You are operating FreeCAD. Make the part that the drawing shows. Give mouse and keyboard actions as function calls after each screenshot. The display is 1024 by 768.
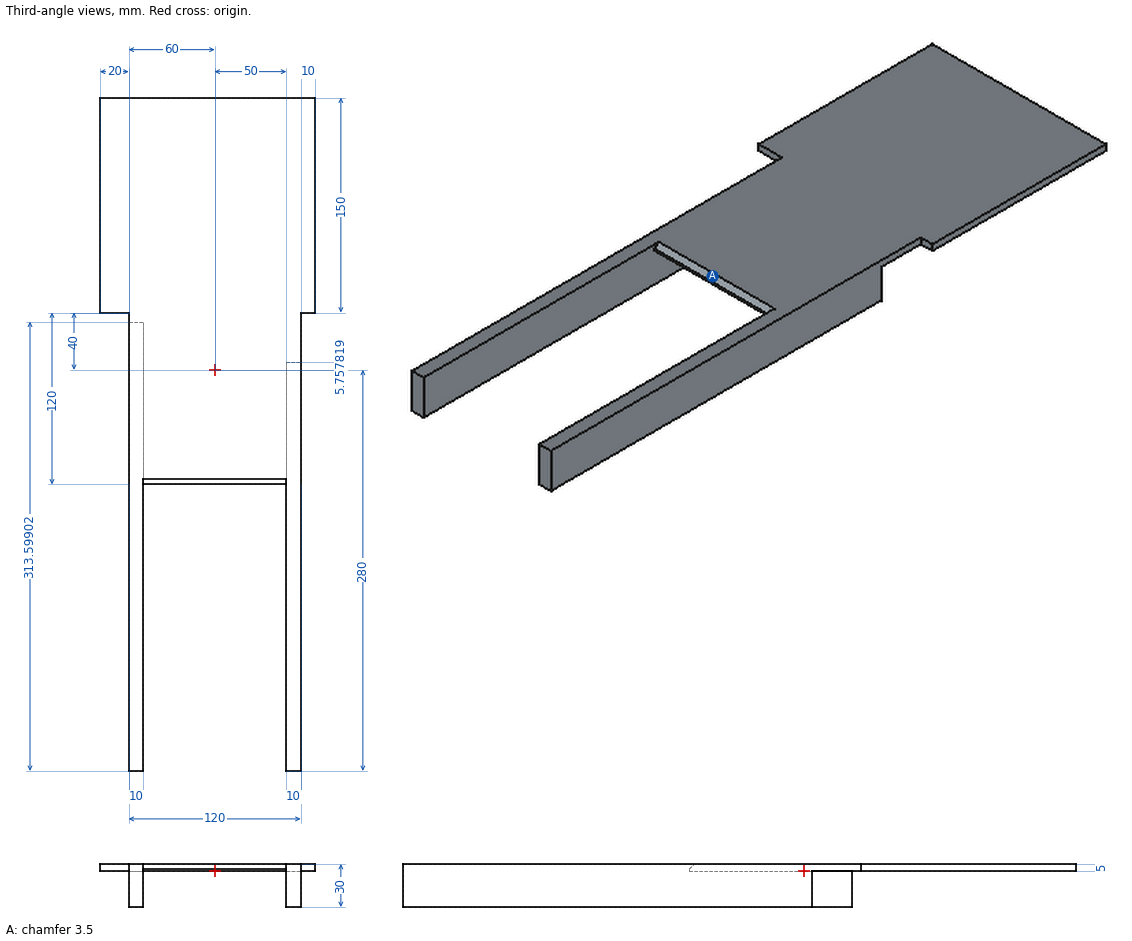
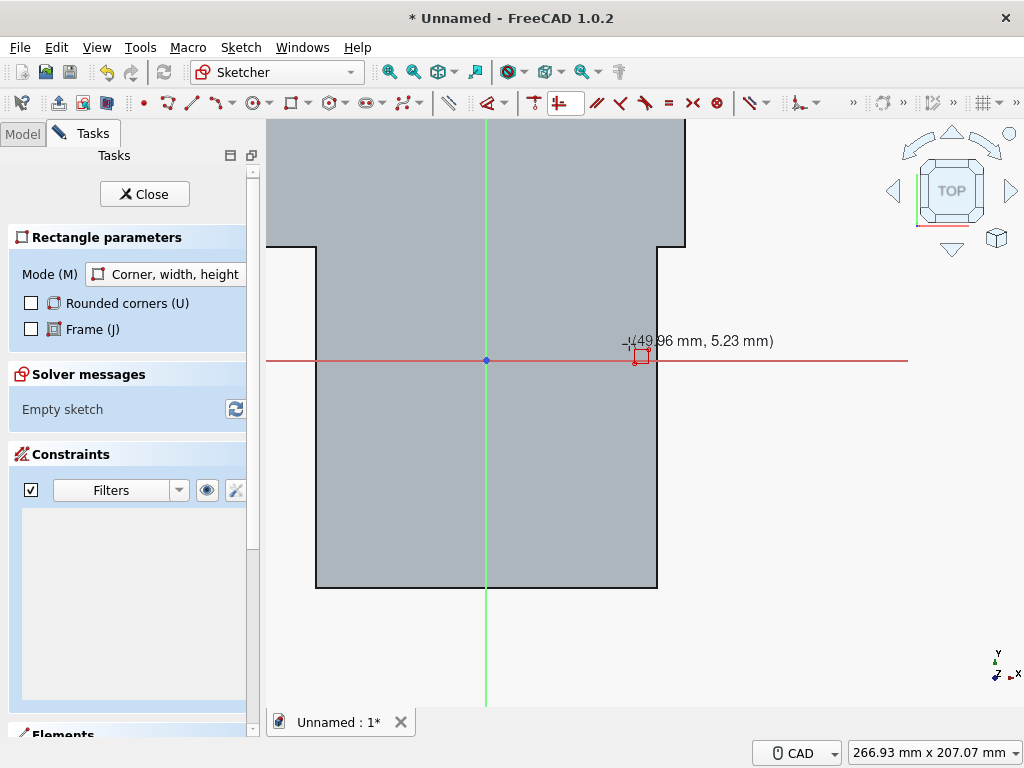
click(628, 345)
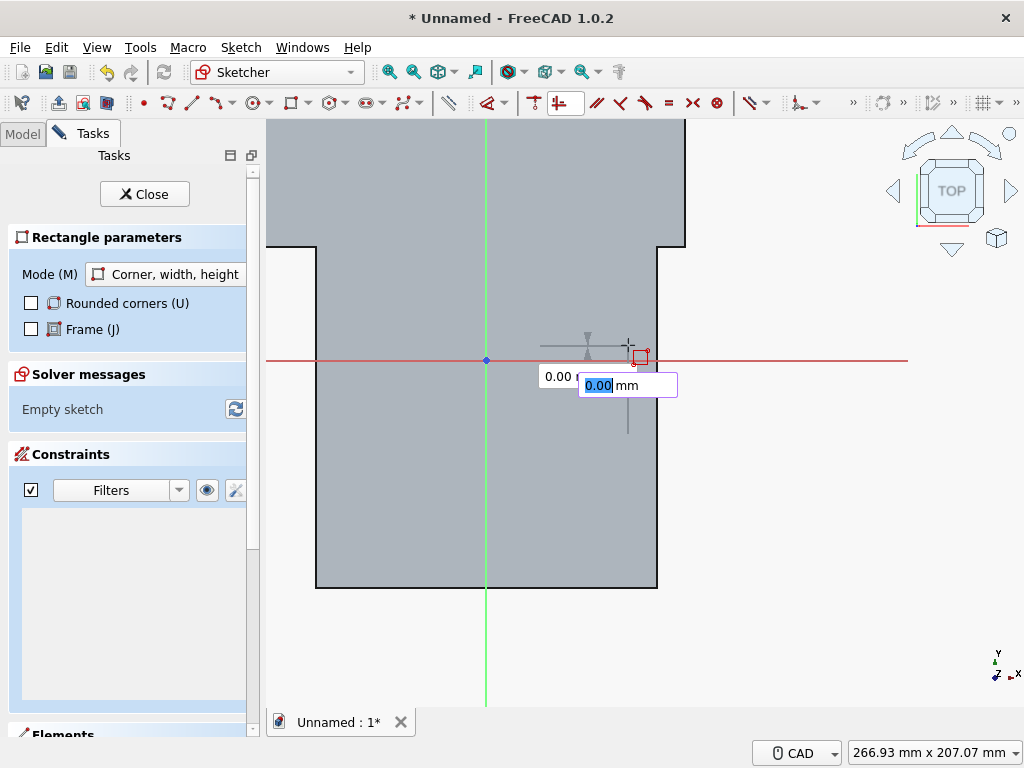
scroll(650, 170, down, 4)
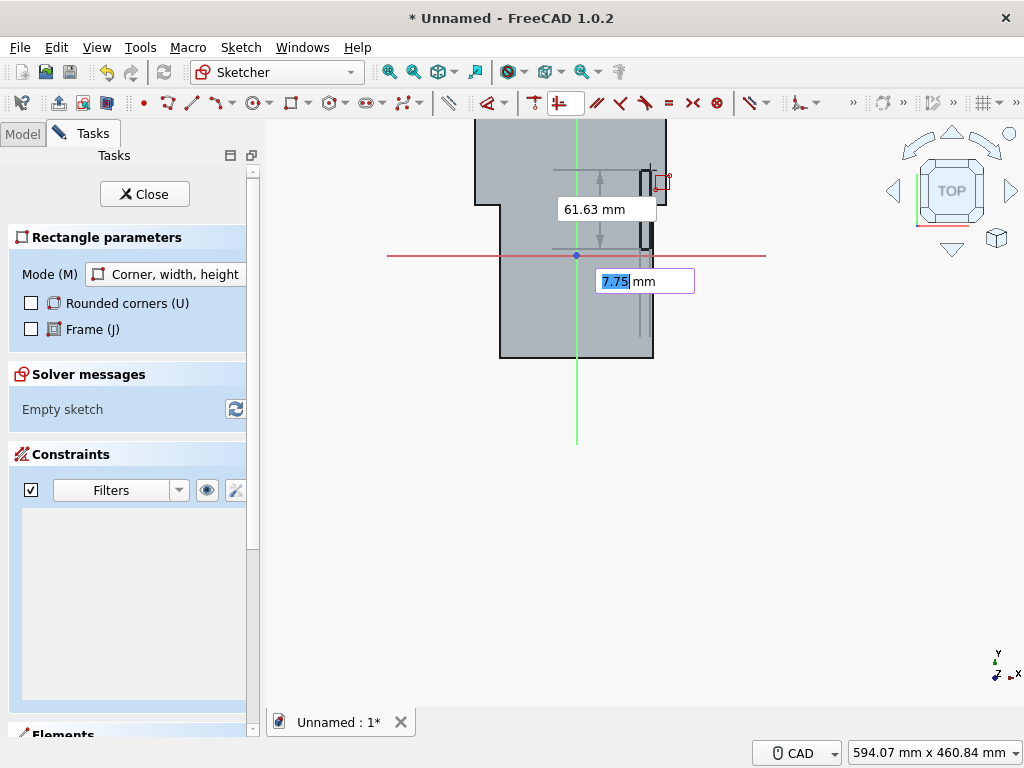
click(653, 613)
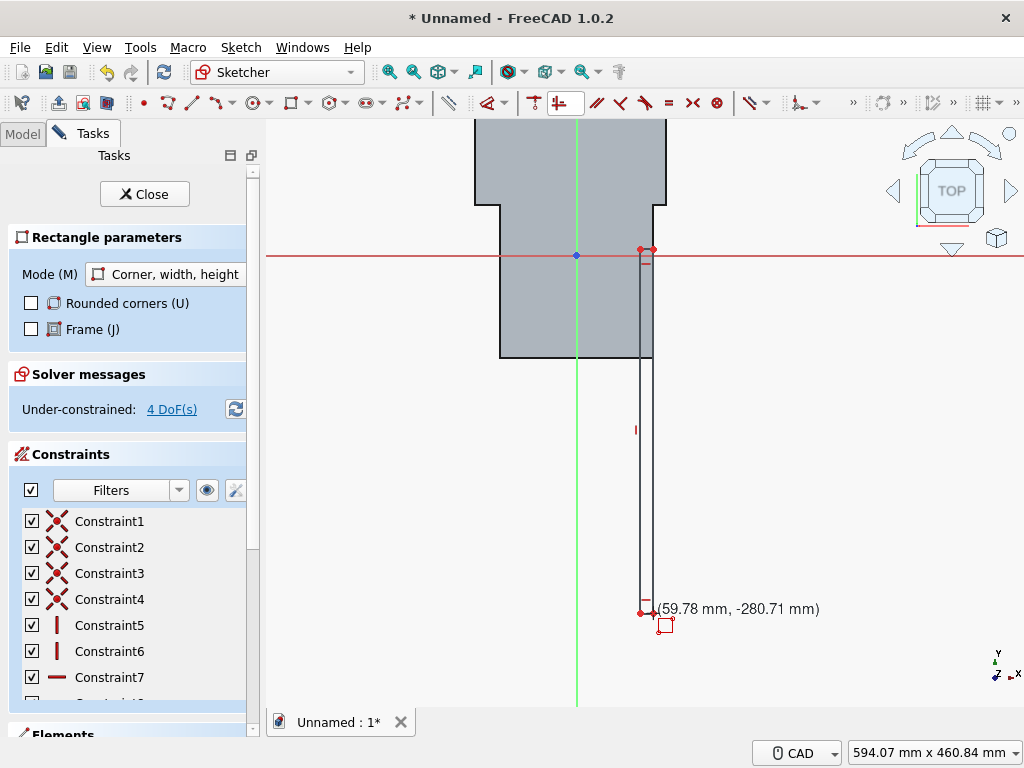
scroll(500, 213, up, 2)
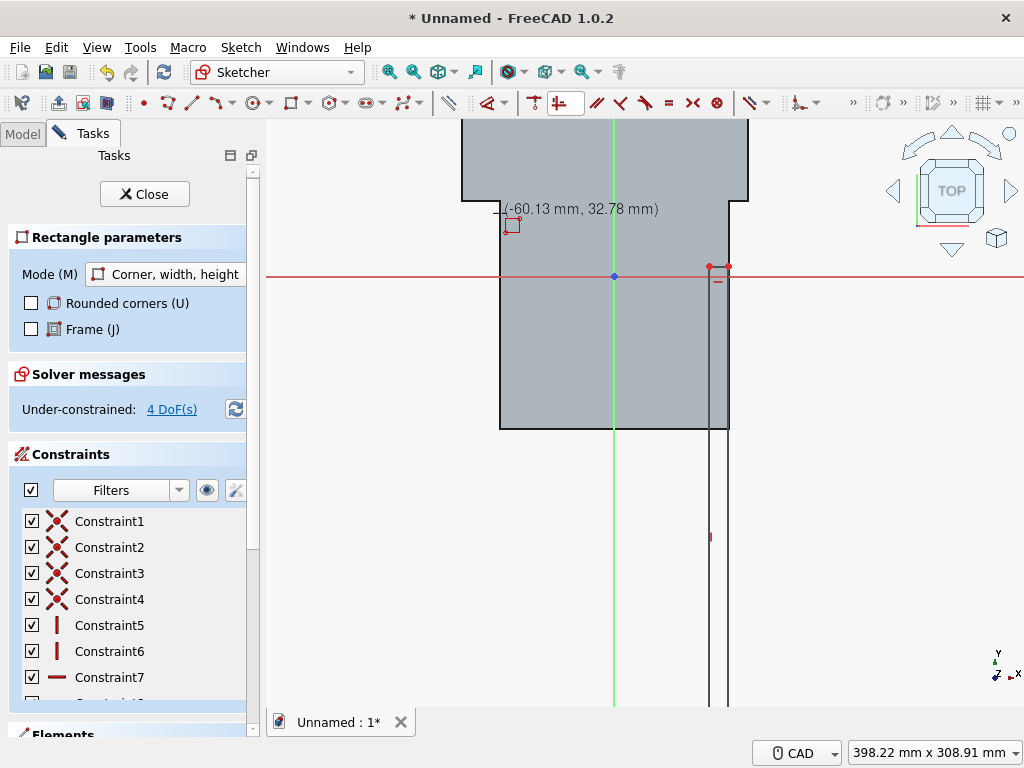
click(500, 213)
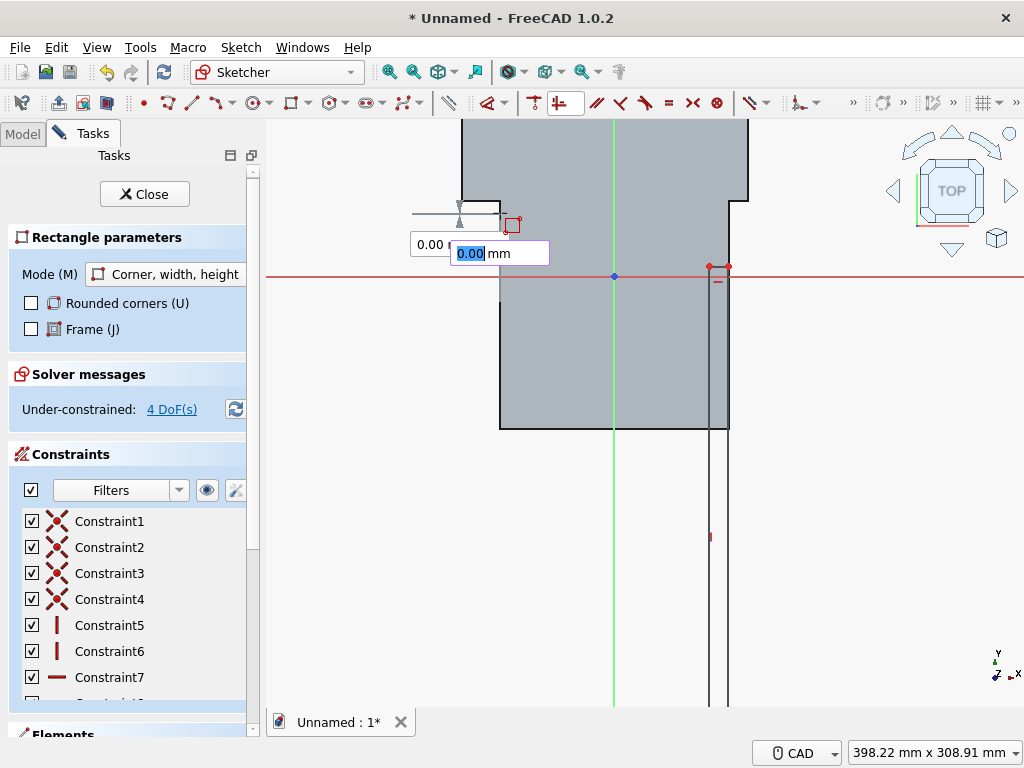
scroll(500, 213, down, 2)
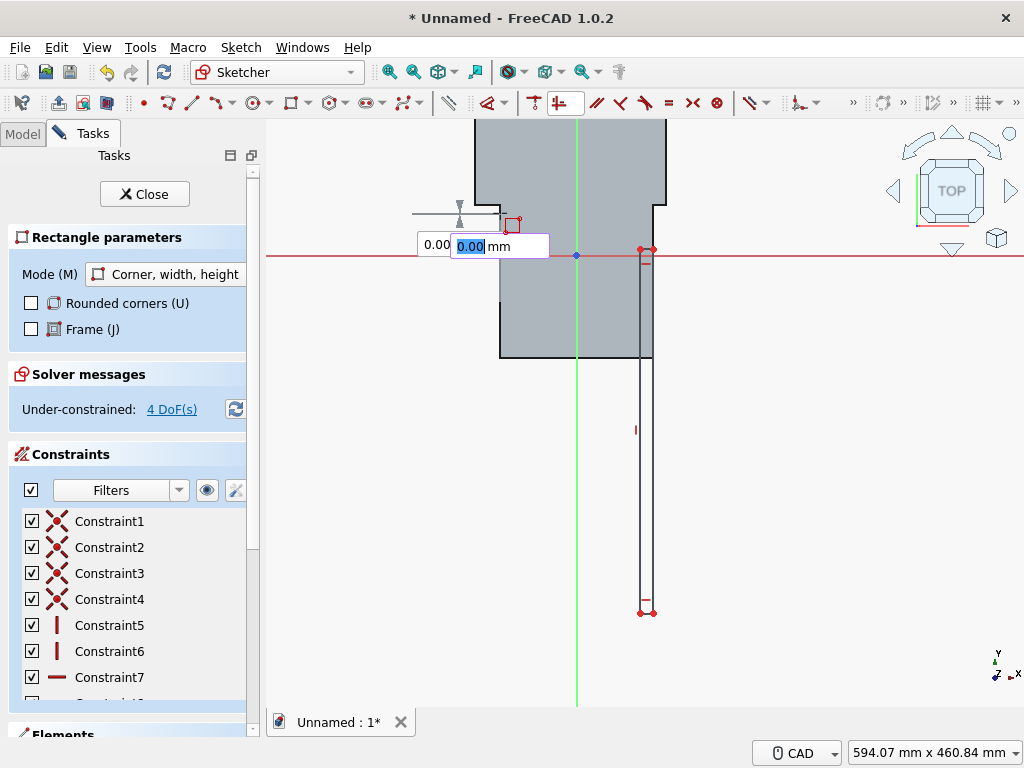
click(513, 613)
key(Escape)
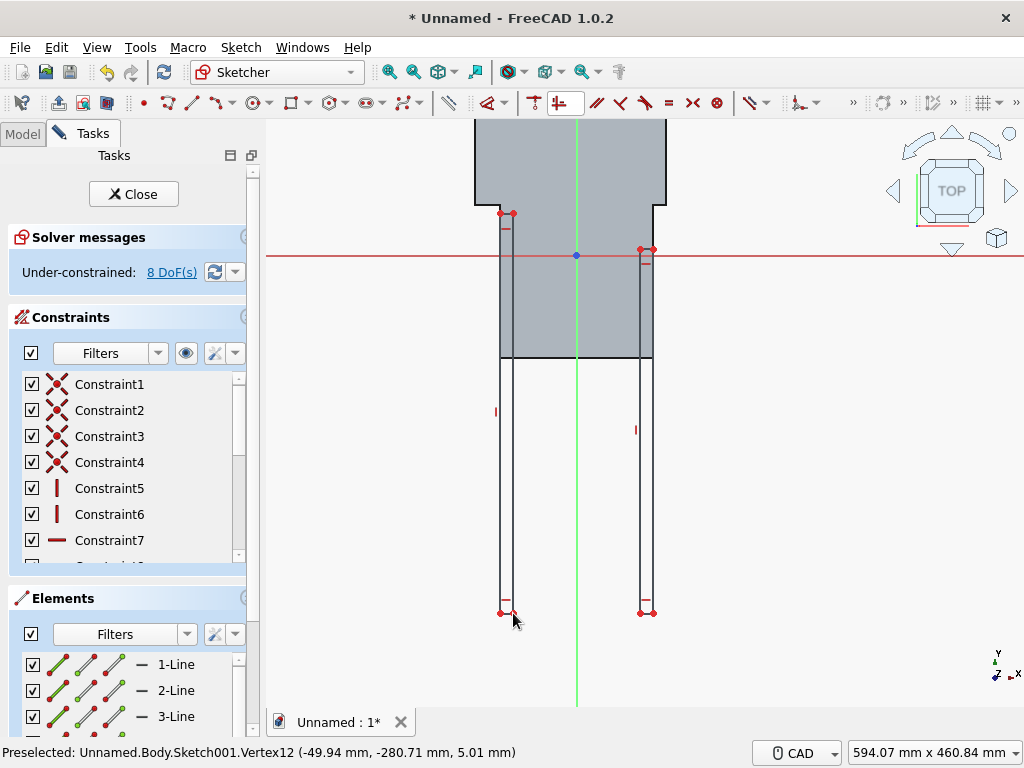
click(488, 104)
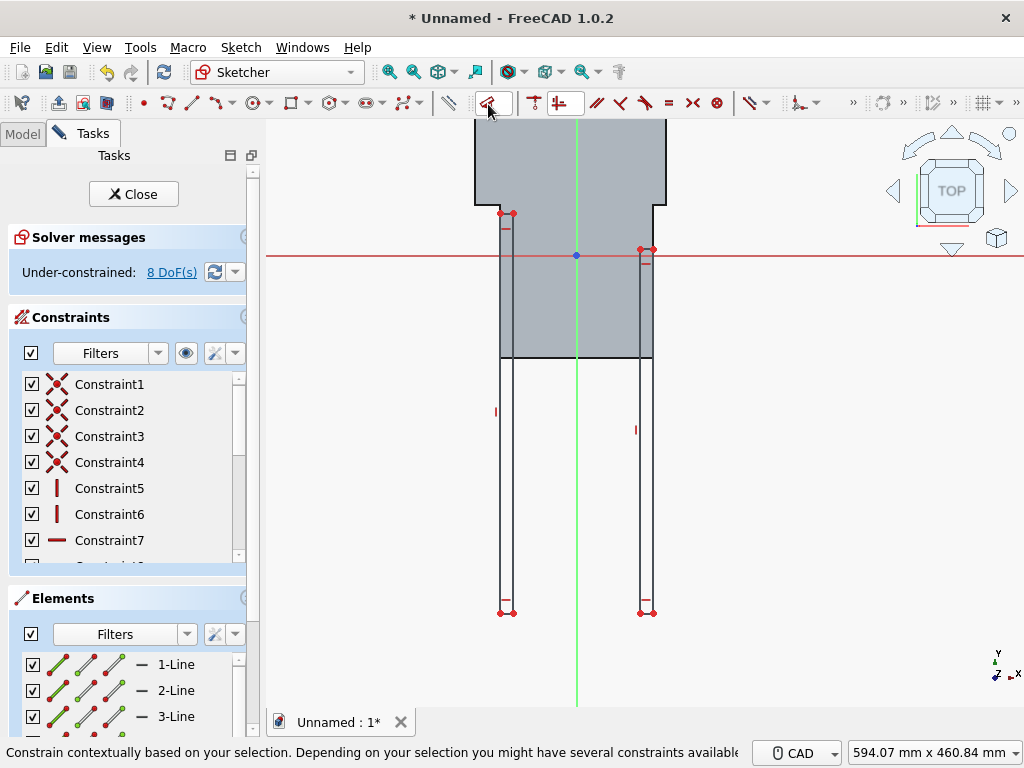
scroll(647, 614, up, 6)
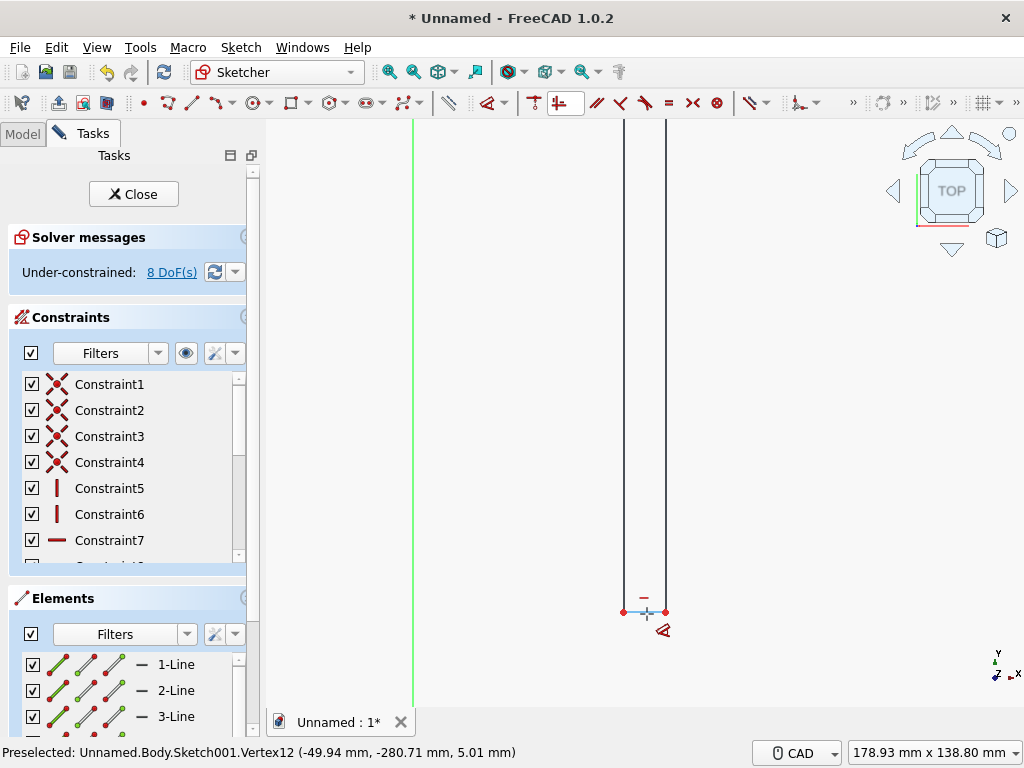
click(645, 612)
click(645, 646)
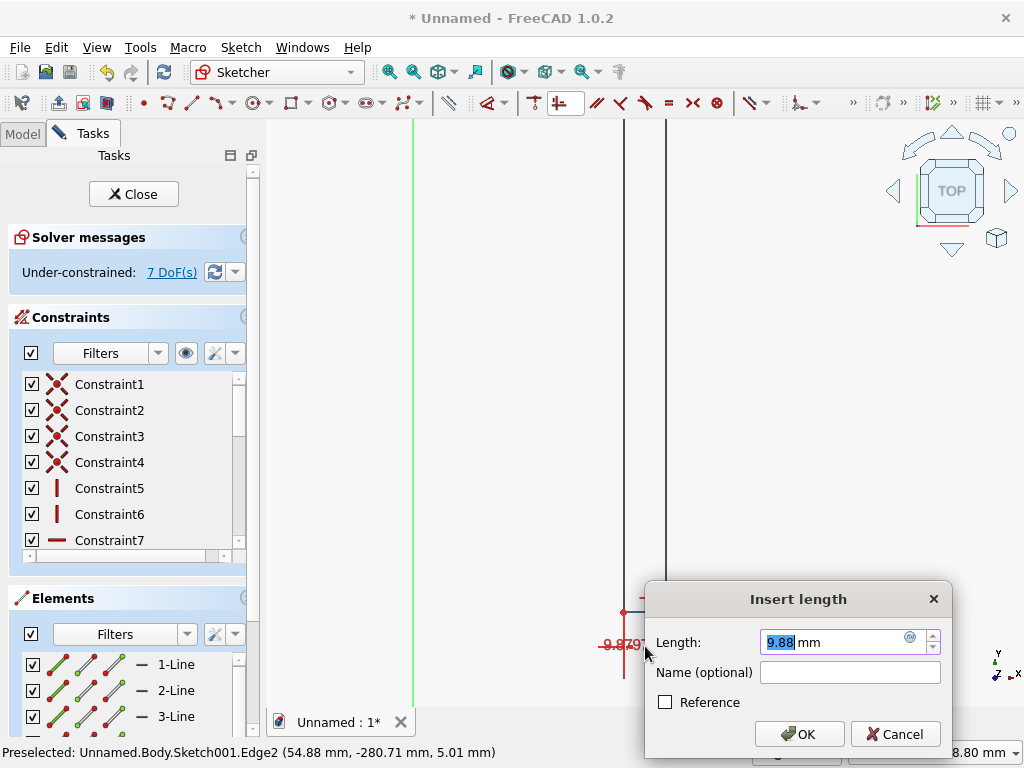
text(10)
key(Return)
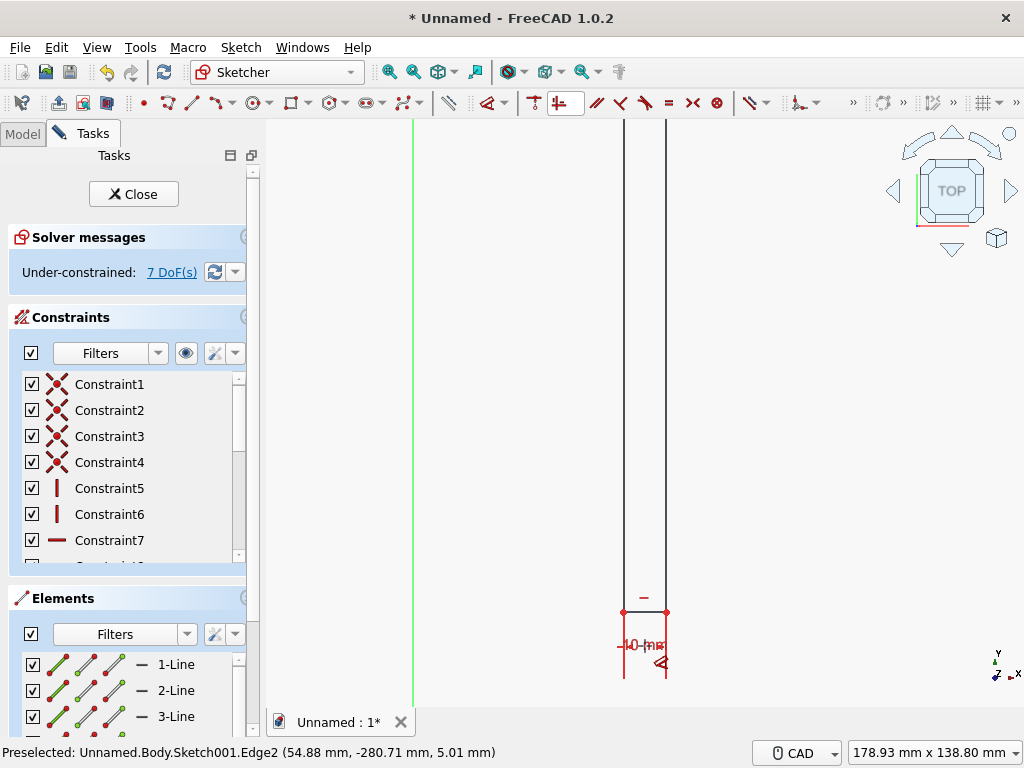
scroll(647, 615, down, 6)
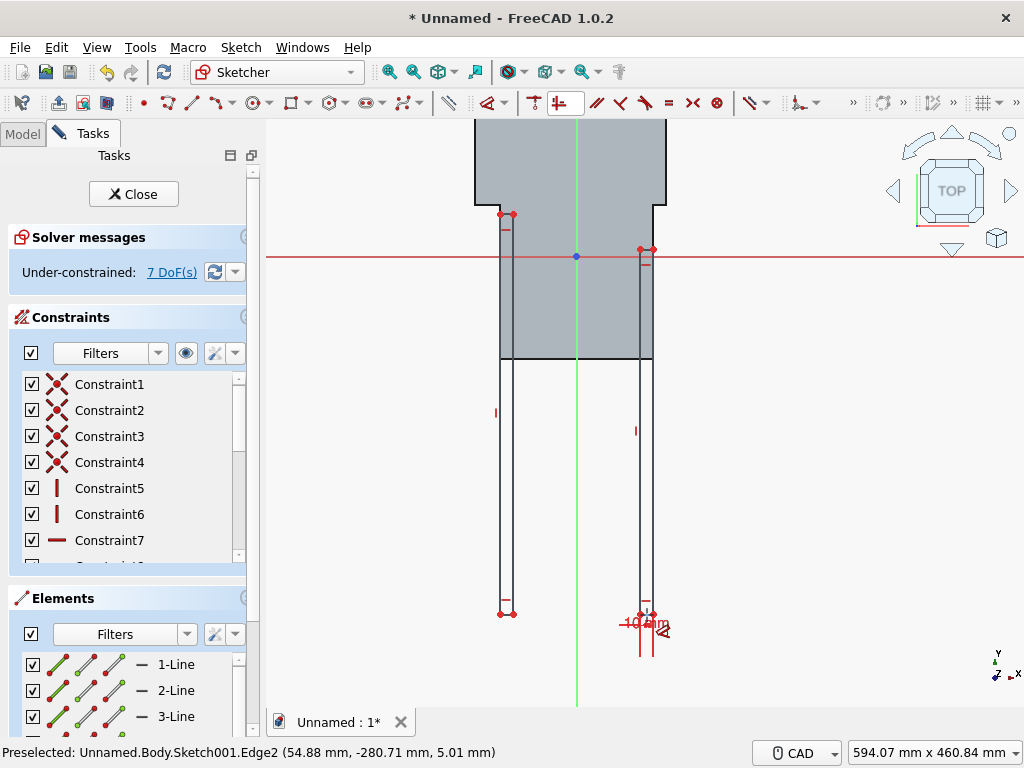
scroll(504, 615, up, 7)